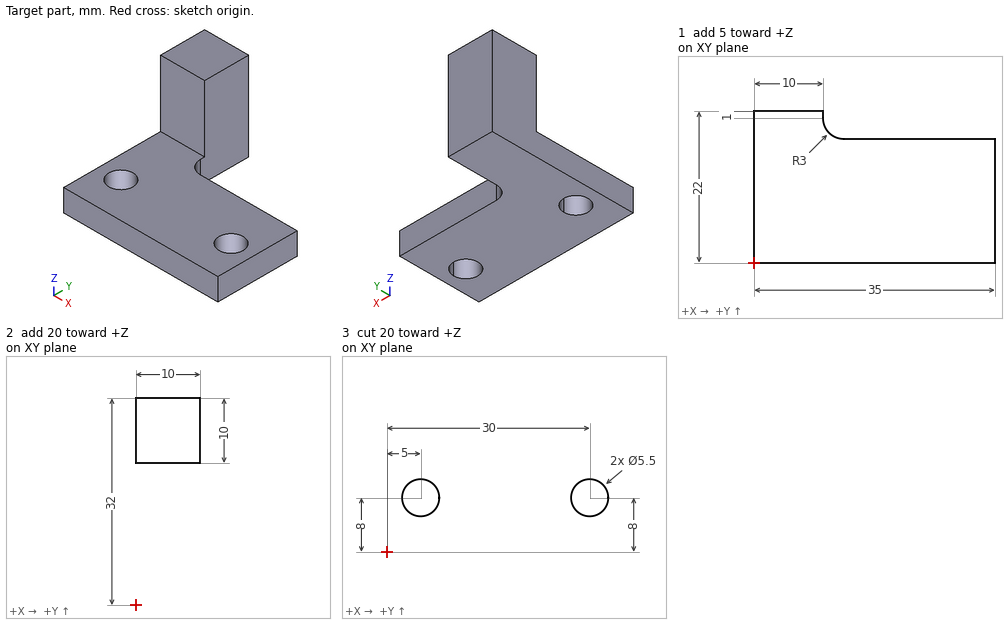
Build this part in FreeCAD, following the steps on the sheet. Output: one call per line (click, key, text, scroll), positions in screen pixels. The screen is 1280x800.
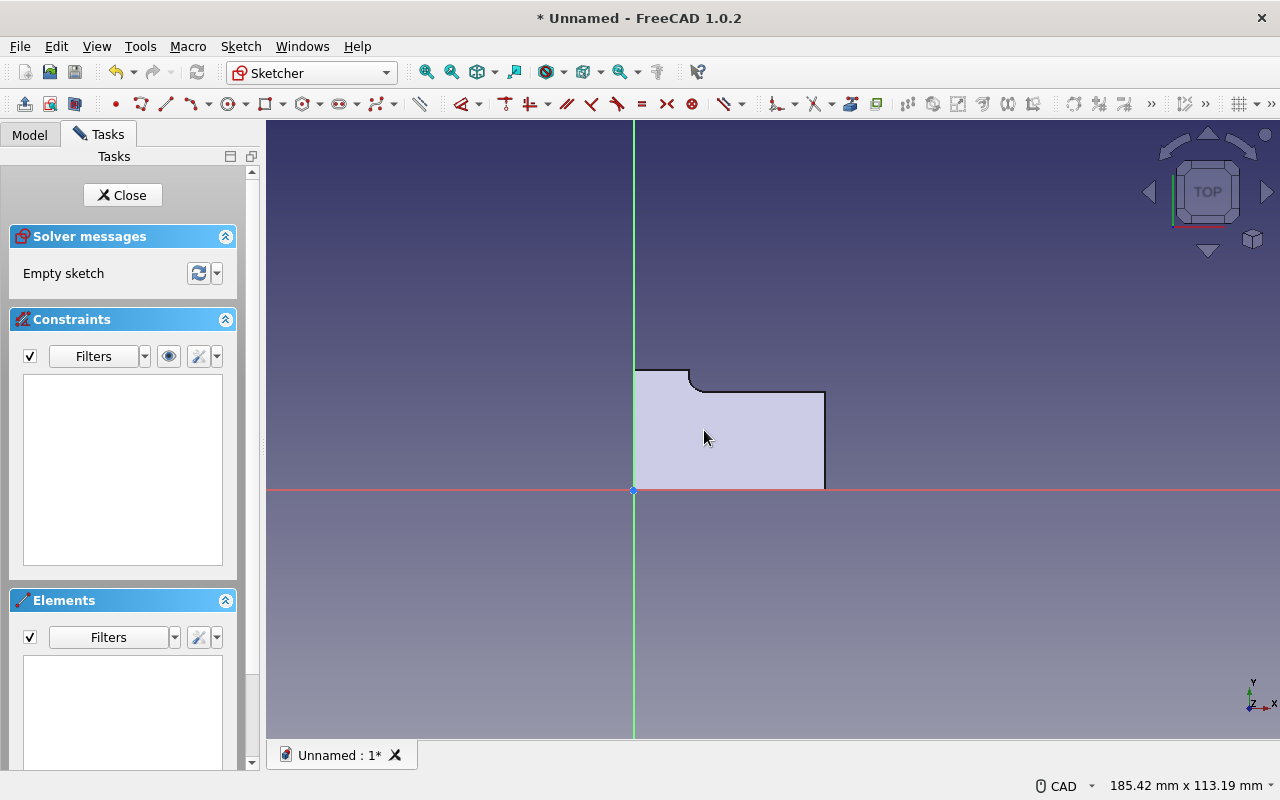
scroll(655, 329, up, 10)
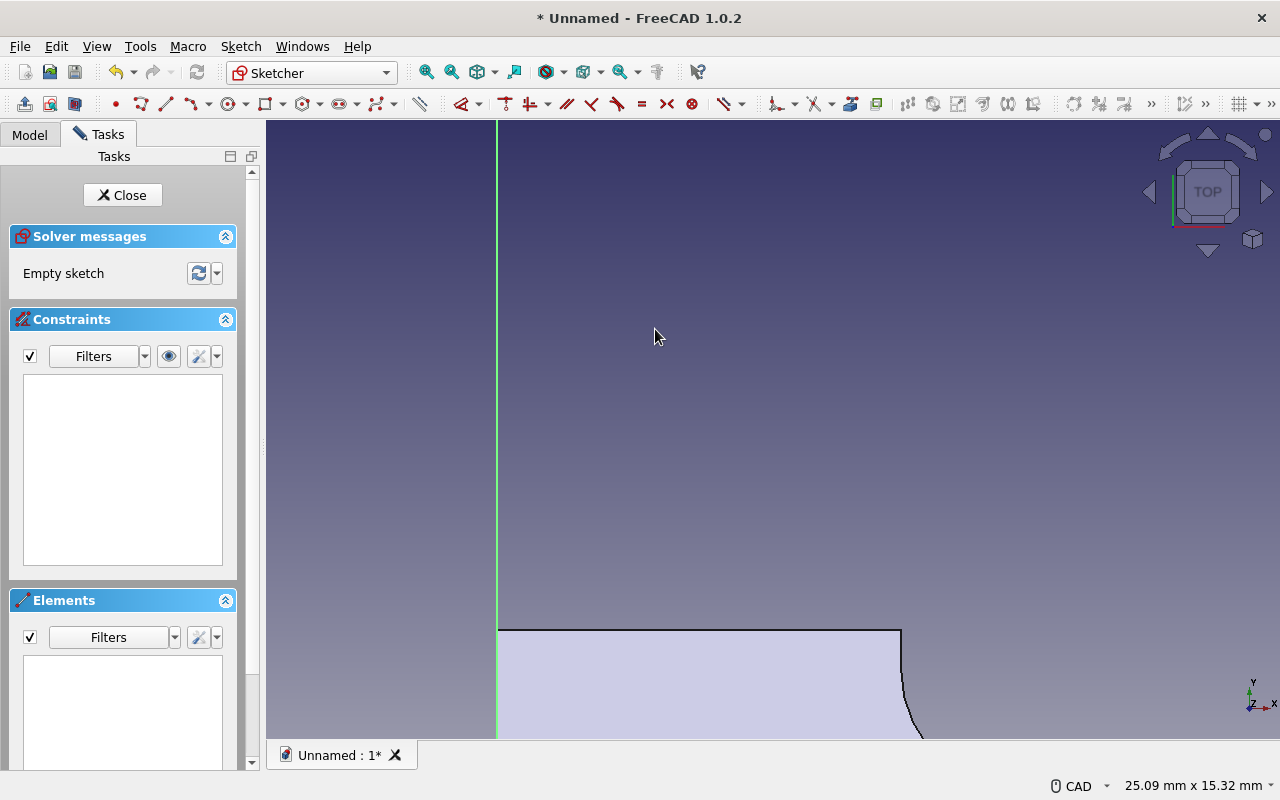
key(g)
key(r)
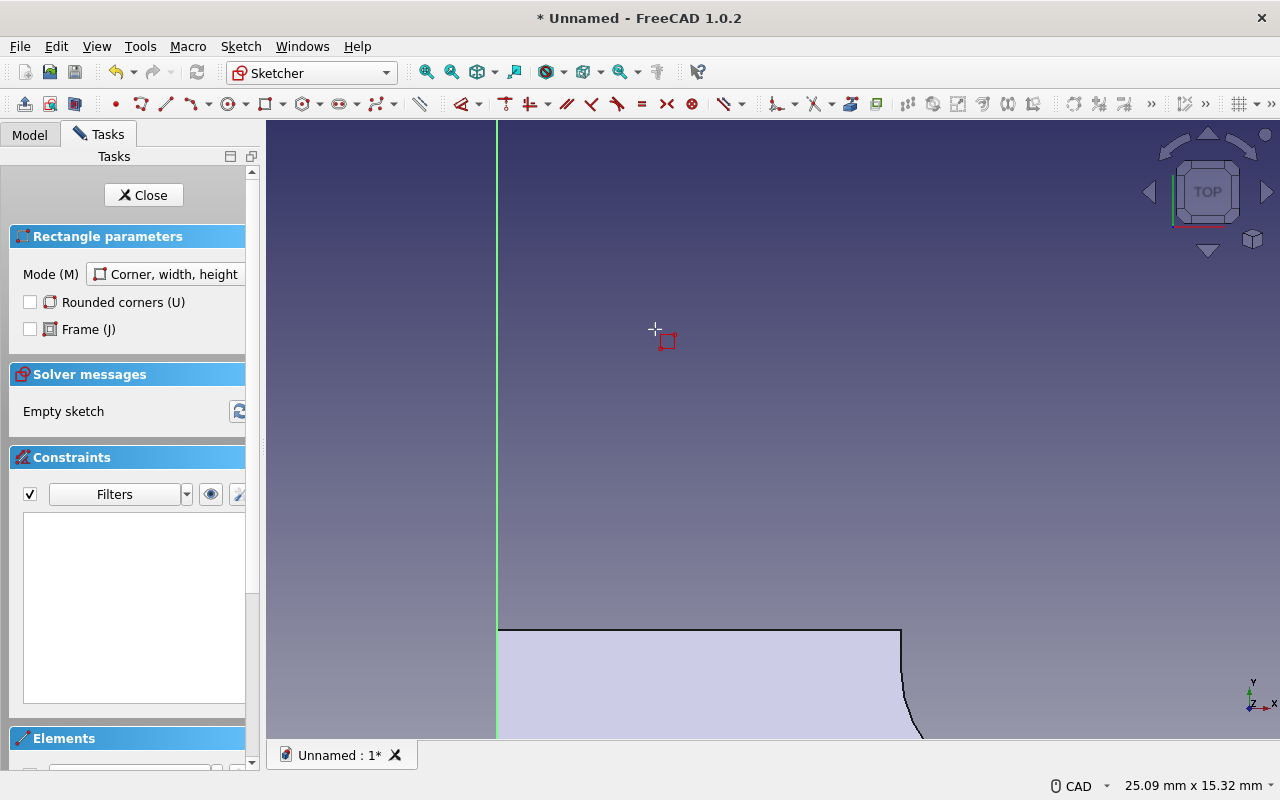
click(497, 226)
move(901, 630)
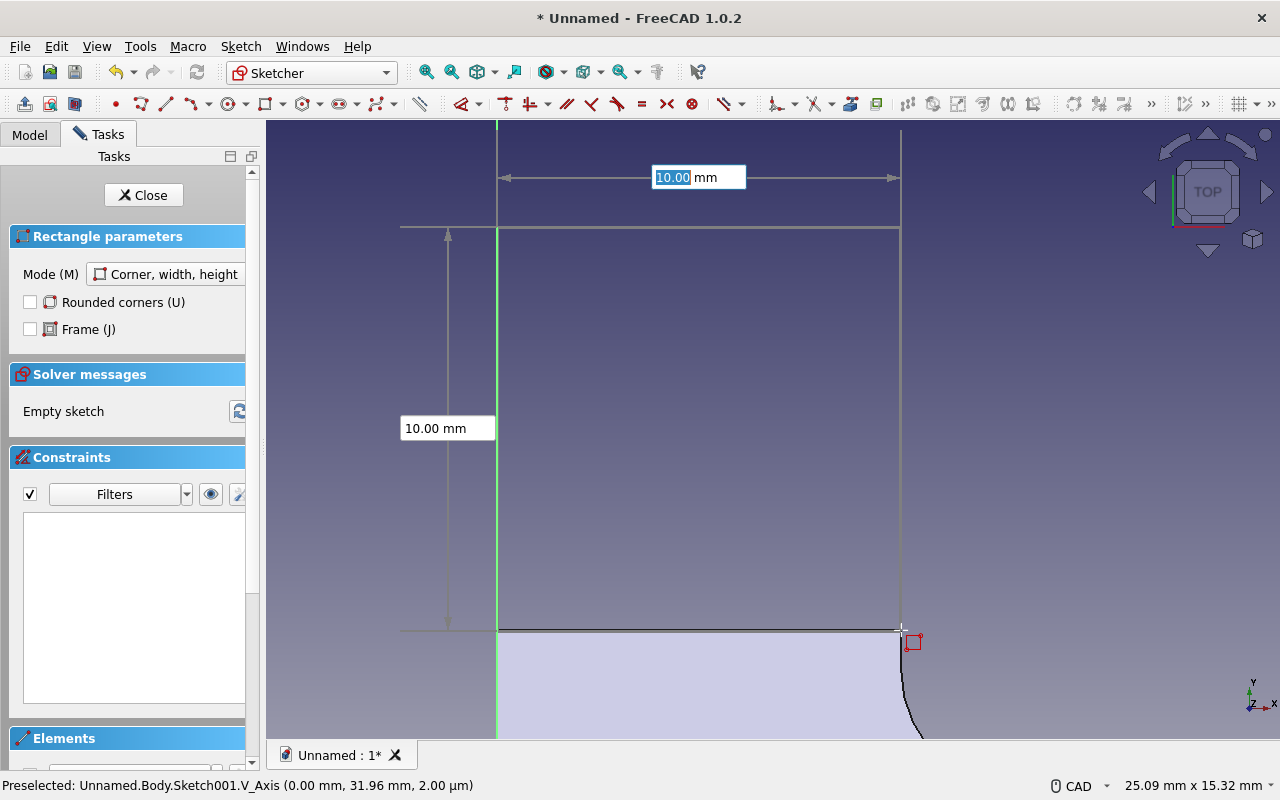
text(10)
key(Tab)
text(10)
key(Return)
key(Escape)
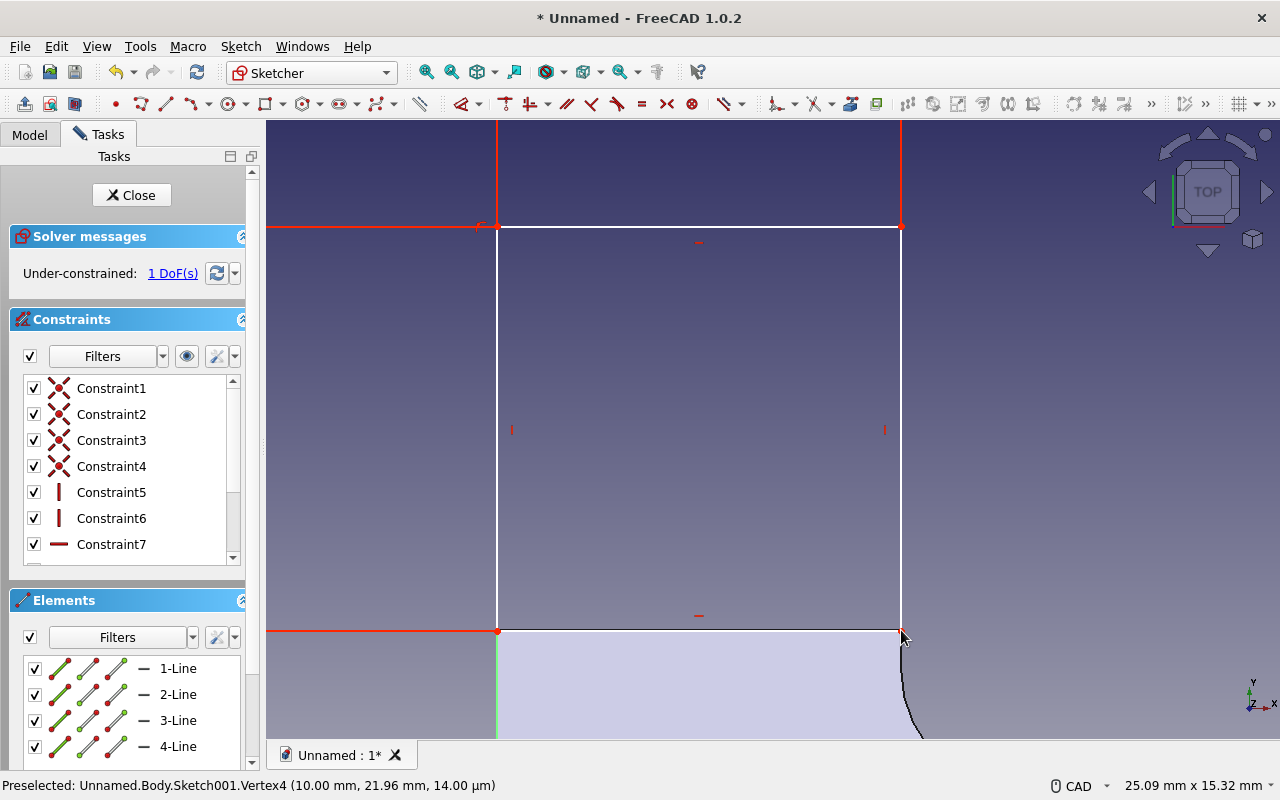
click(460, 104)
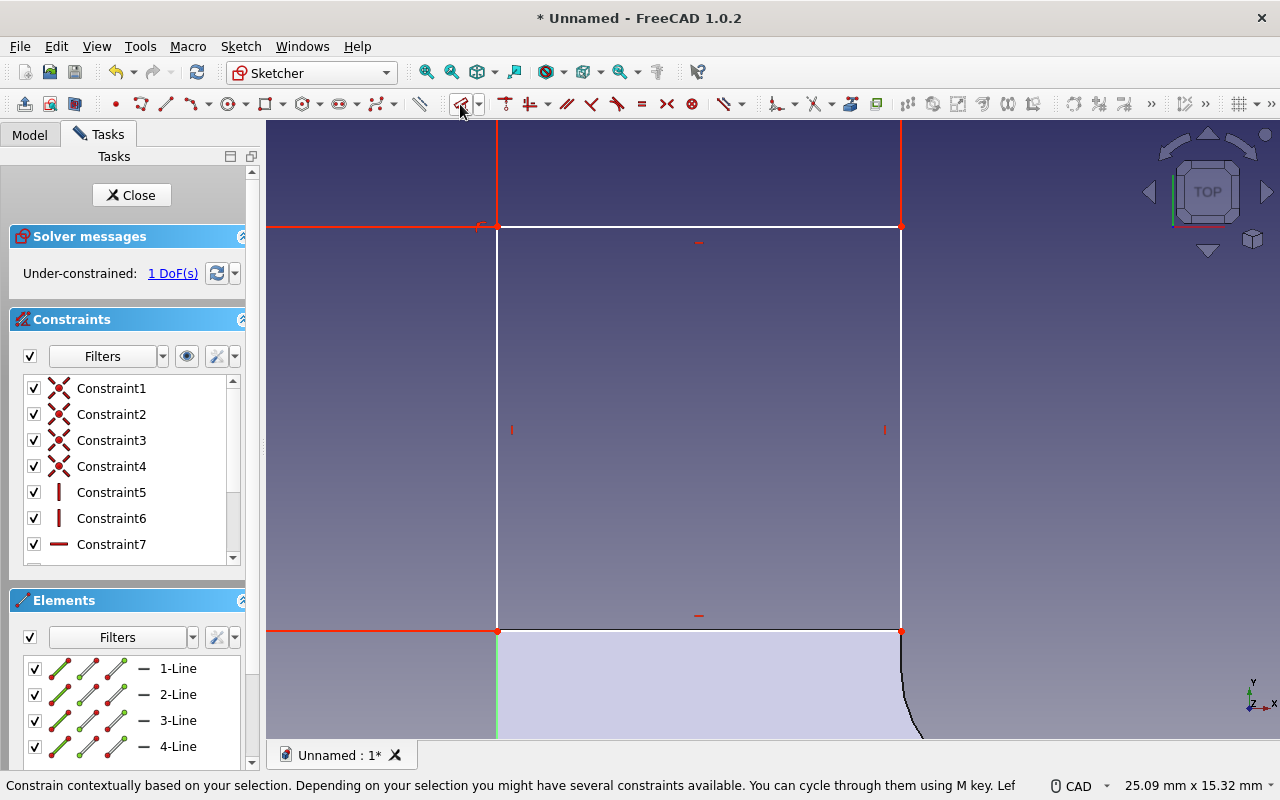
click(497, 227)
click(463, 469)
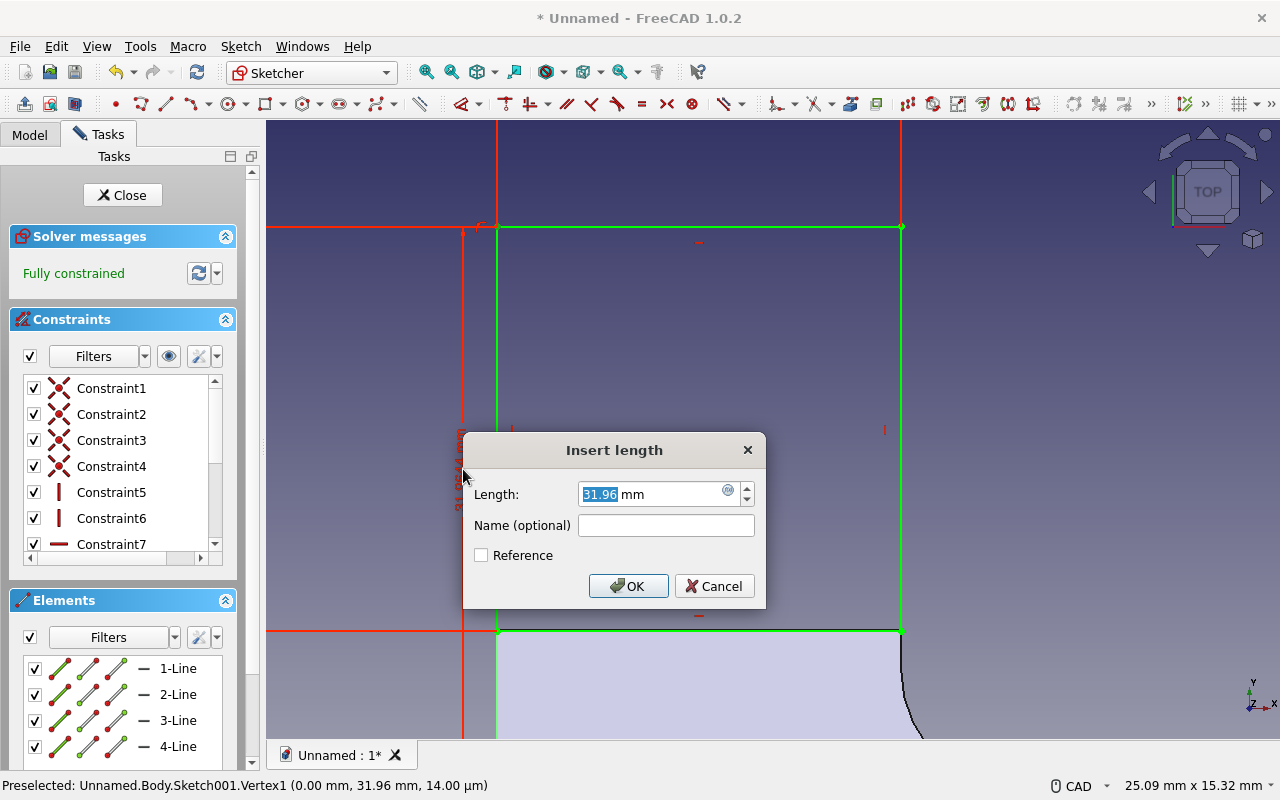
text(32)
key(Return)
key(Escape)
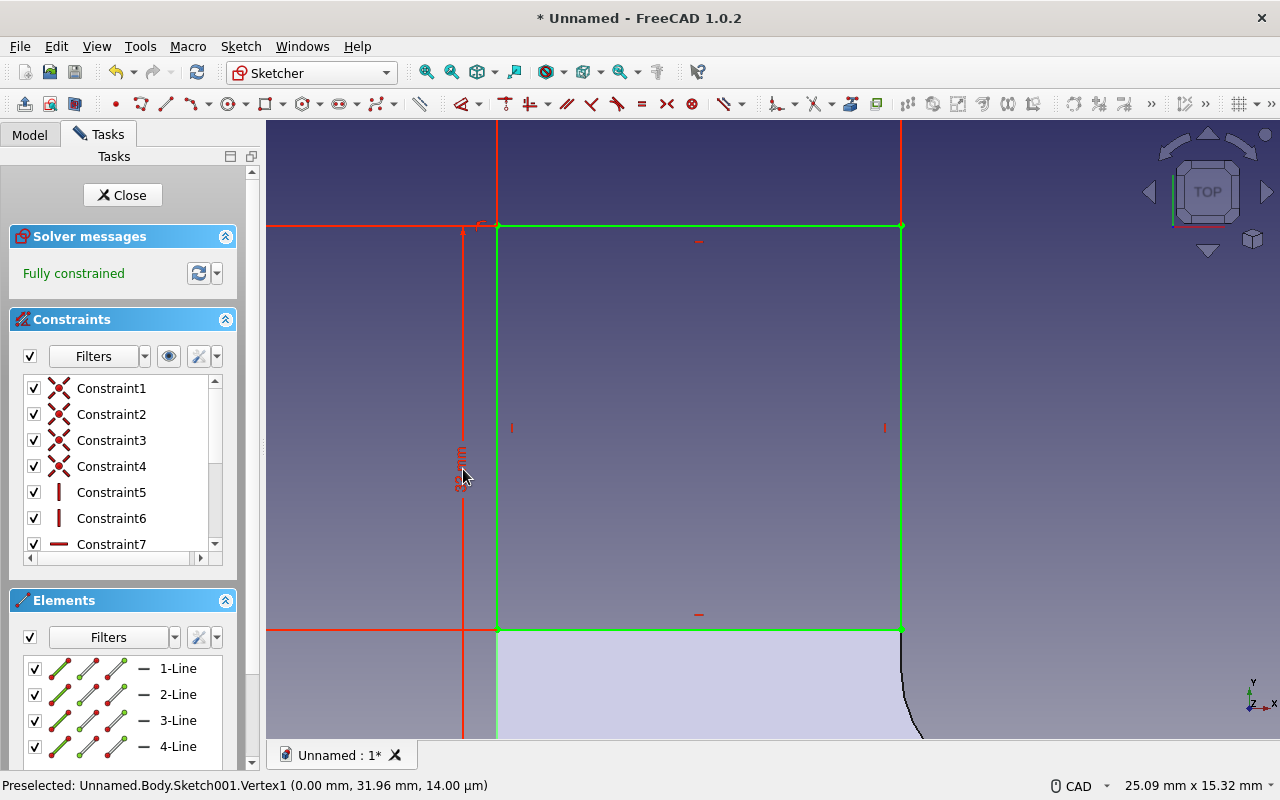
click(123, 195)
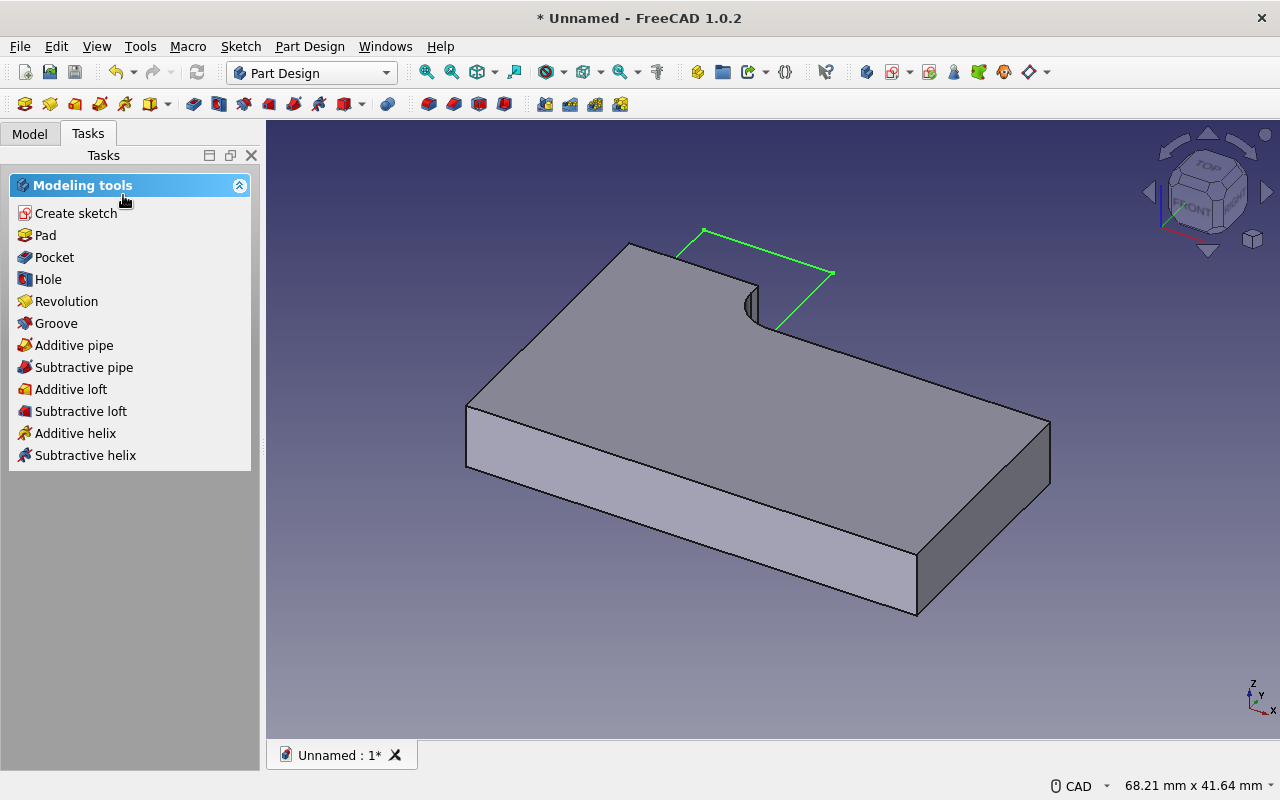
click(25, 104)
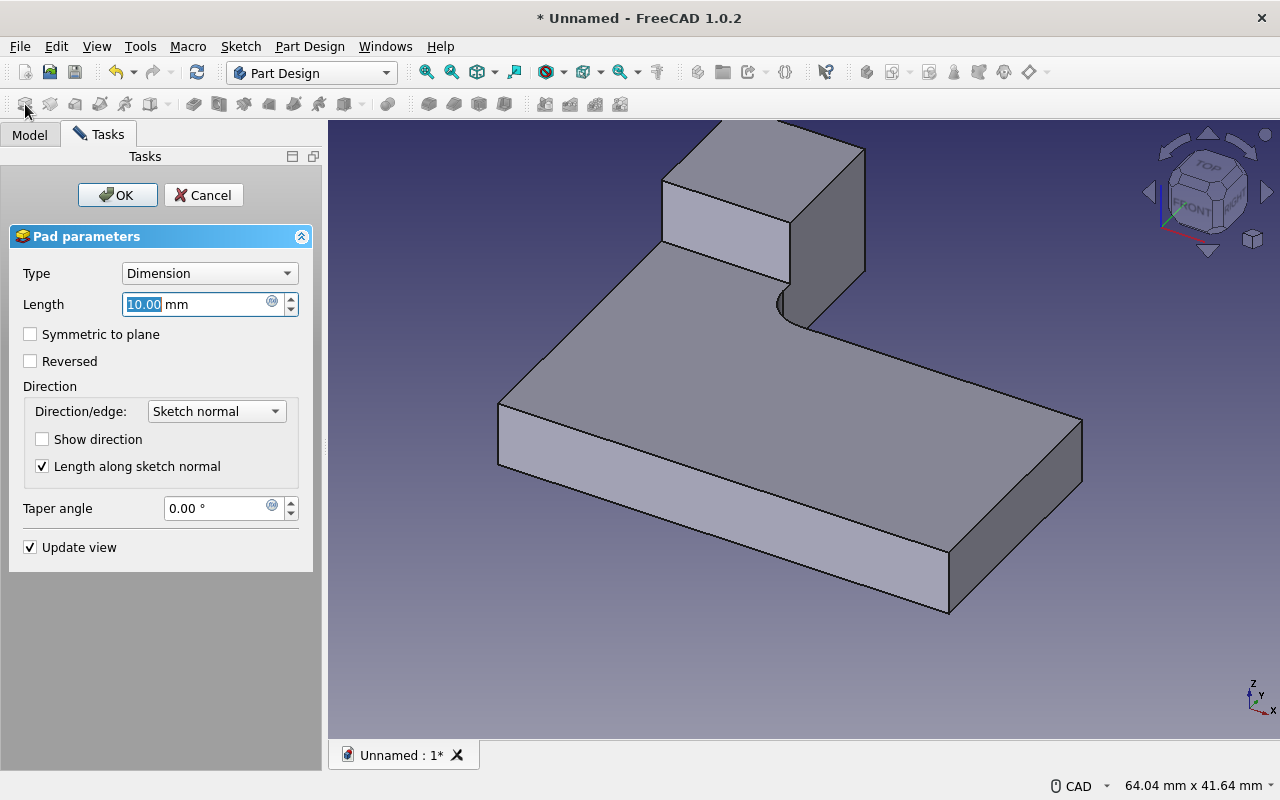
text(20)
key(Tab)